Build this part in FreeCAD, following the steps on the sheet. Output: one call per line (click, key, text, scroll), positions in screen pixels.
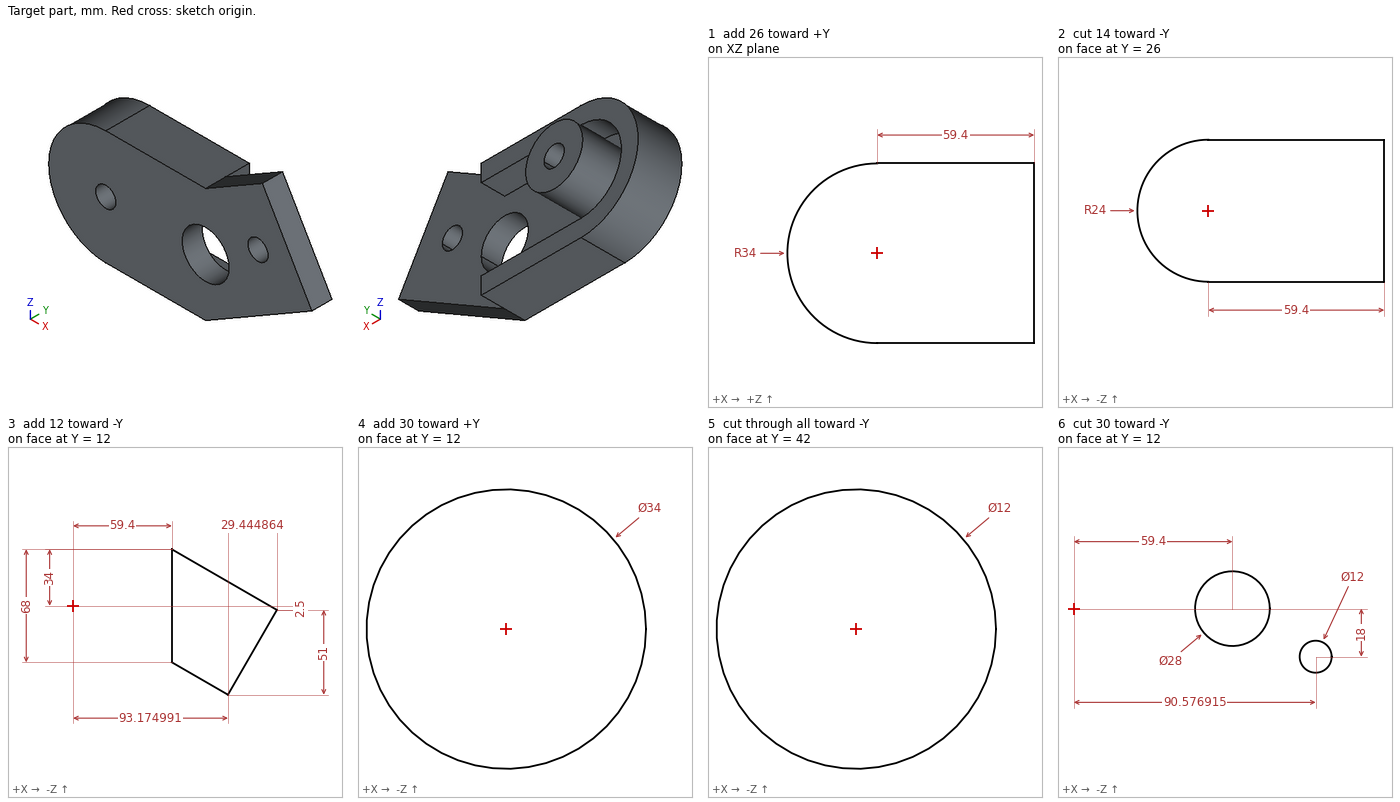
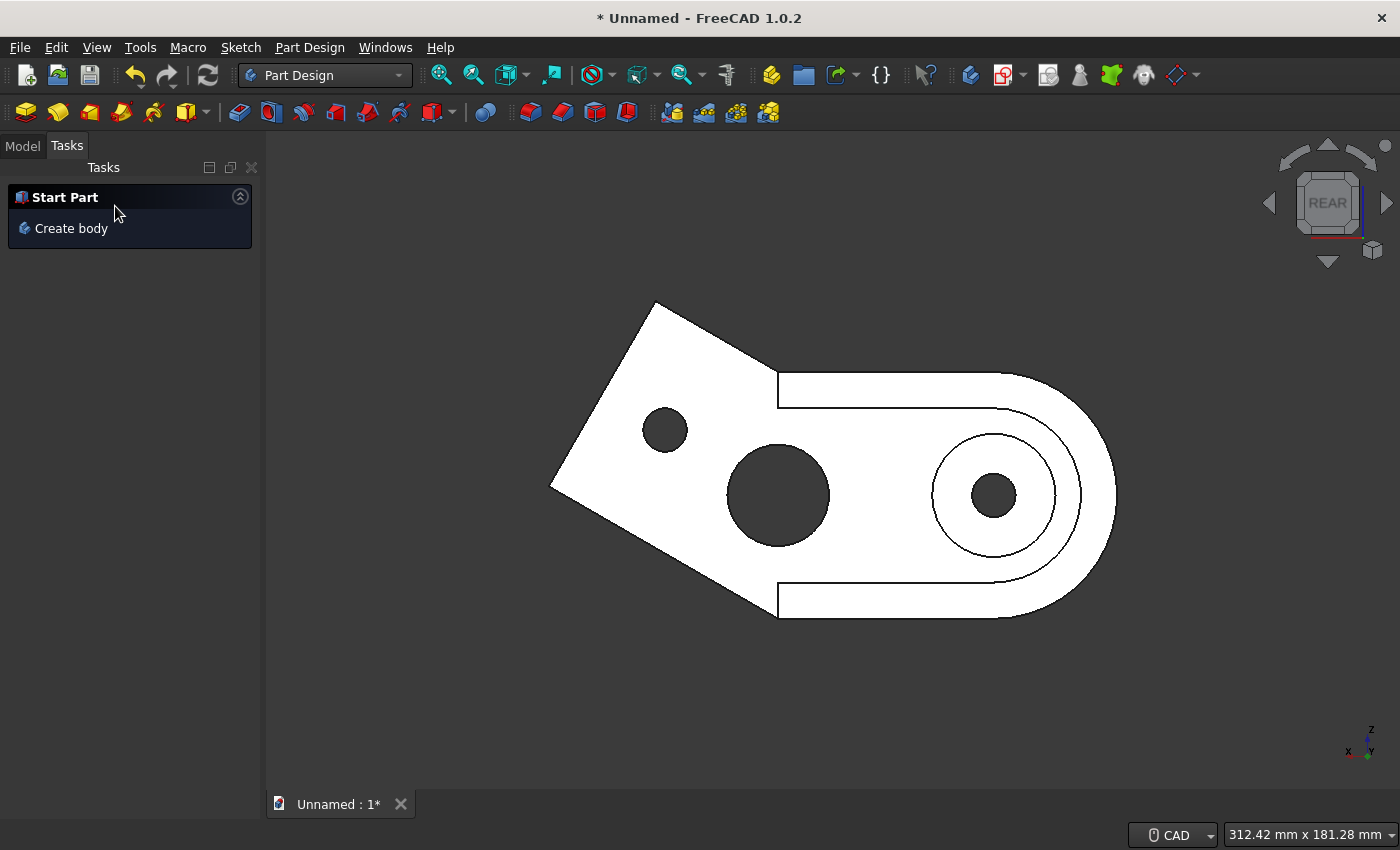
key(0)